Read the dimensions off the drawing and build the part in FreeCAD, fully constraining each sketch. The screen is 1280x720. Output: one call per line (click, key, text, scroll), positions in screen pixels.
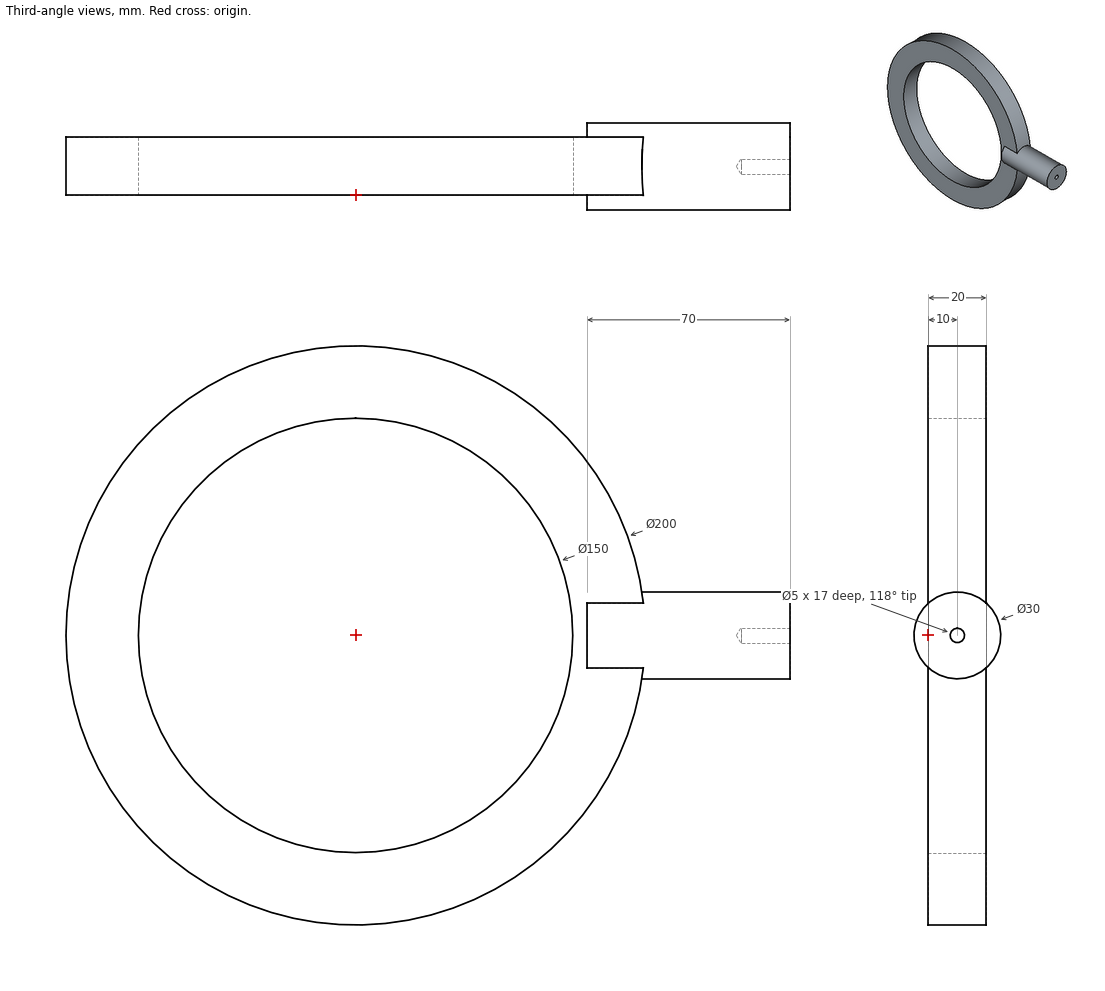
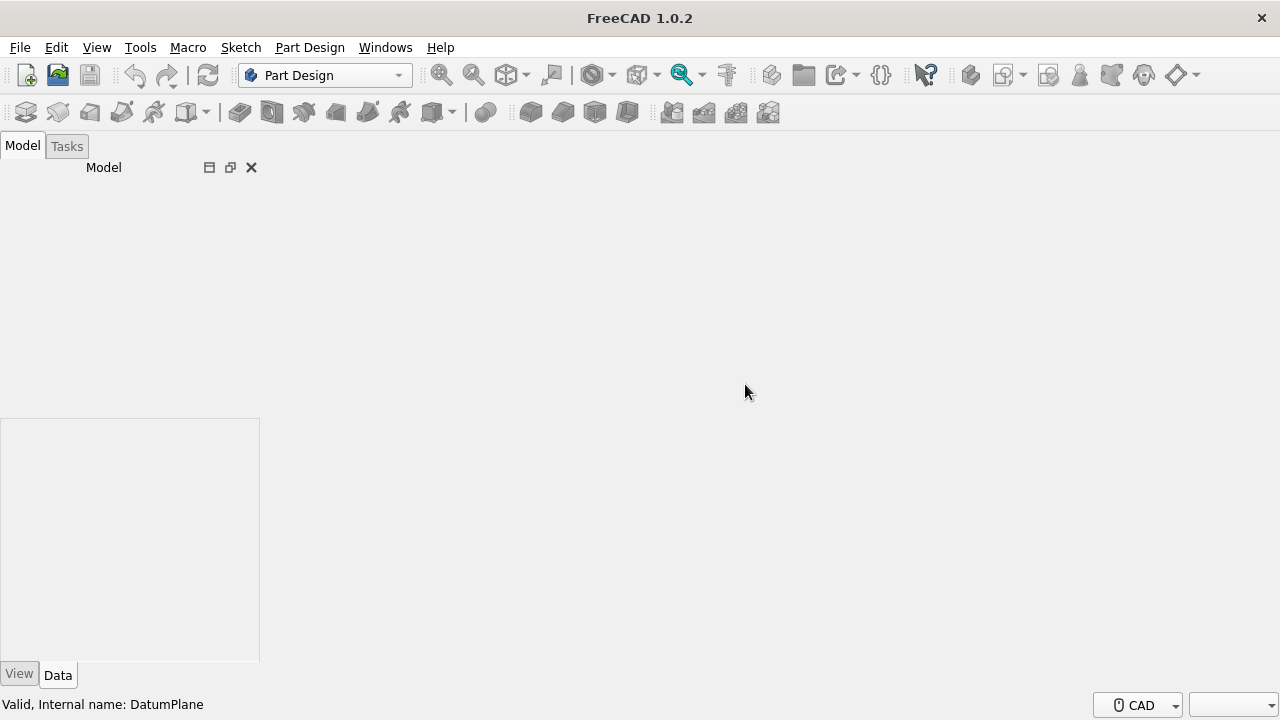
key(ctrl+n)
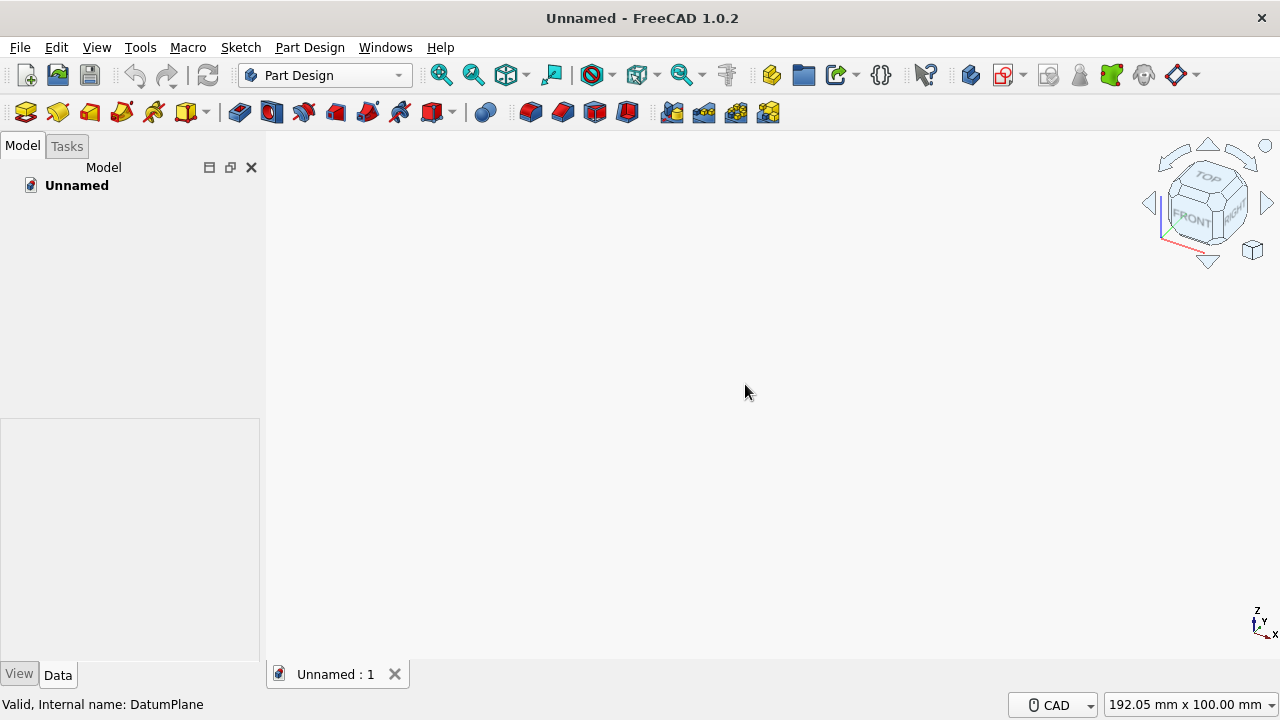
click(1004, 76)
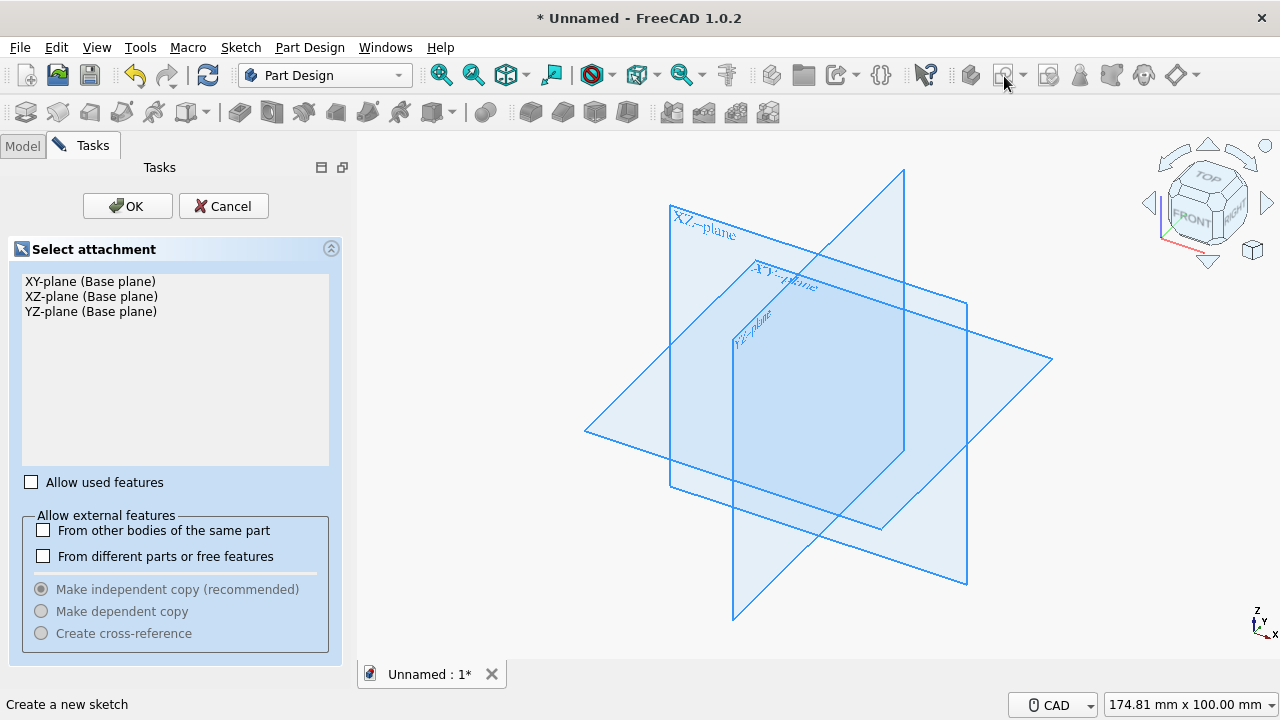
click(82, 296)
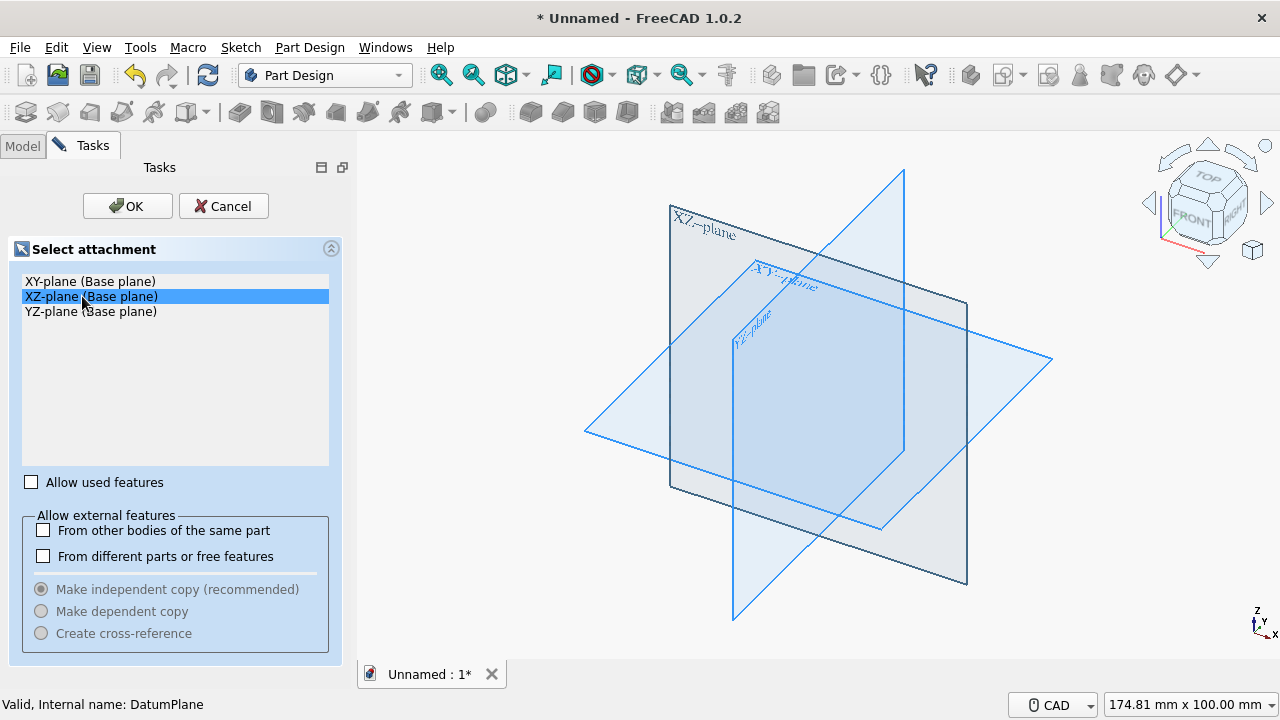
click(128, 206)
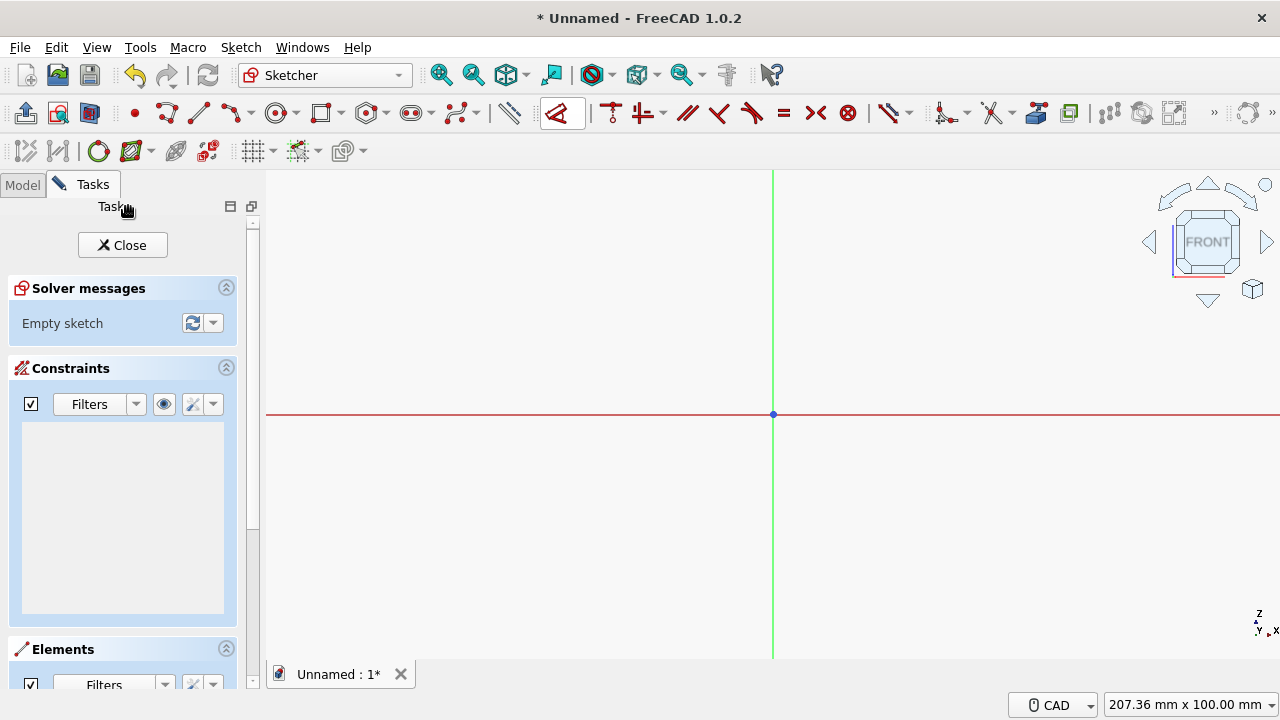
scroll(675, 414, down, 6)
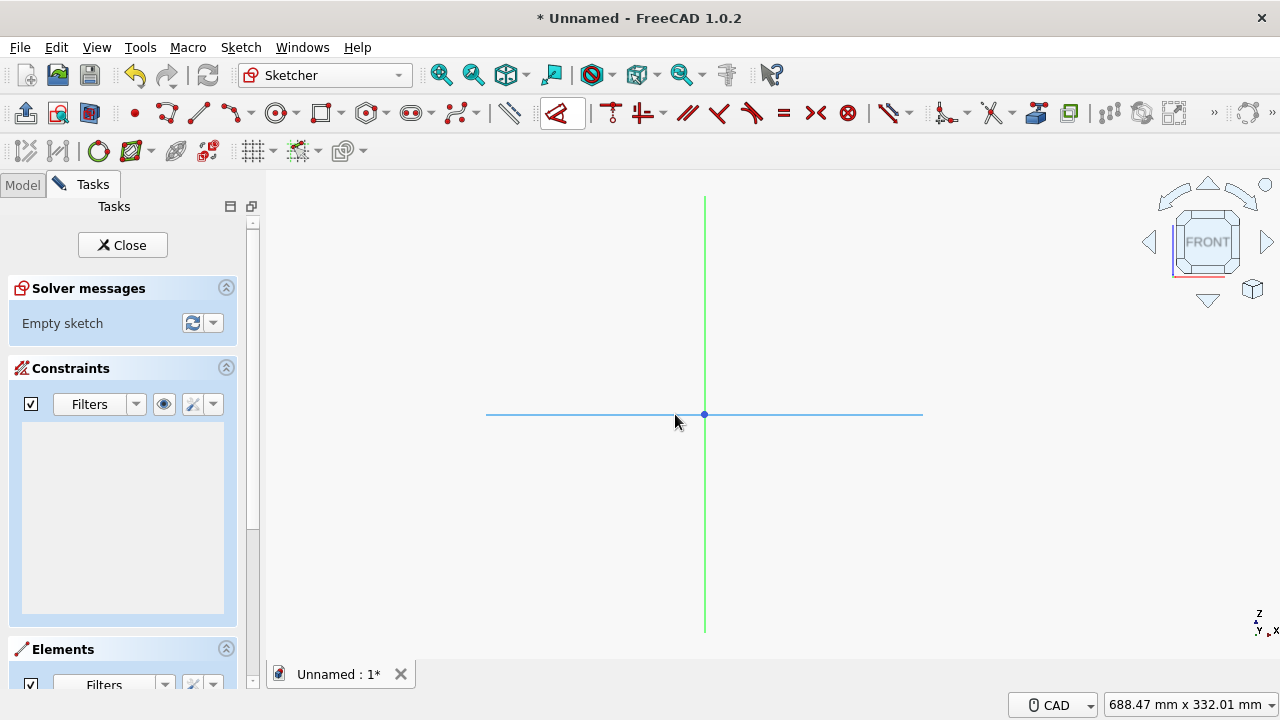
key(g)
key(c)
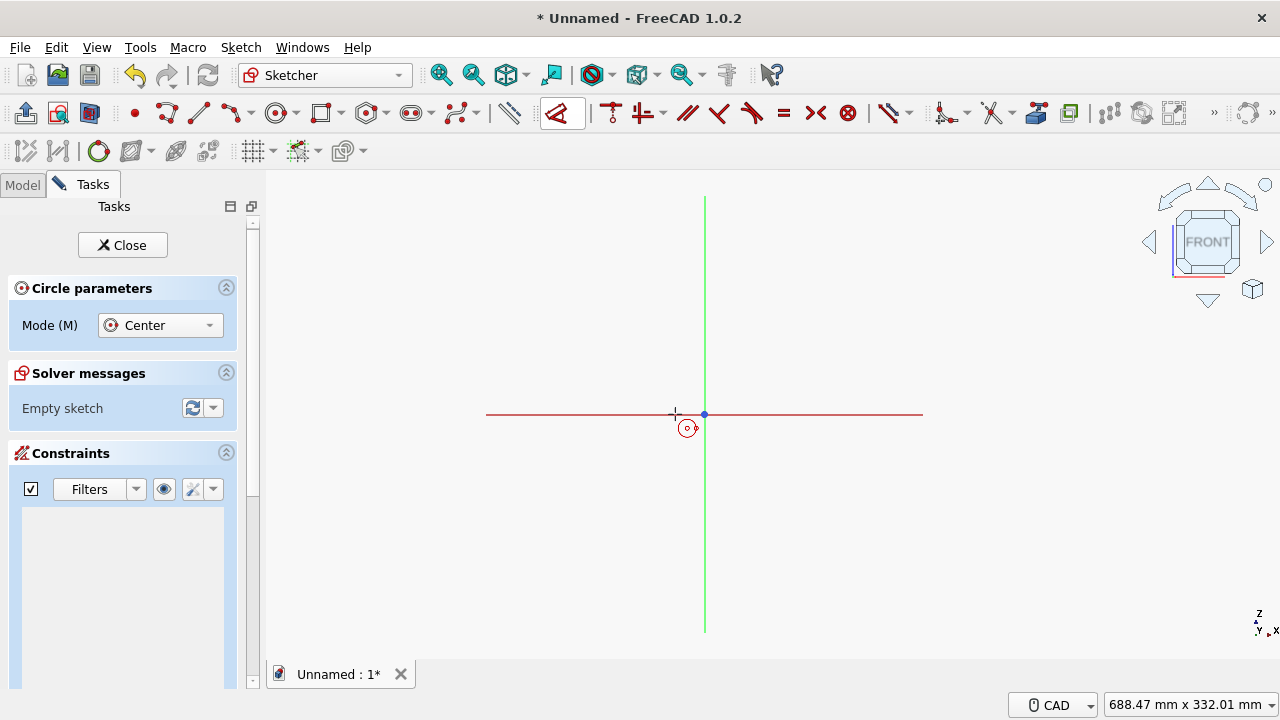
click(705, 414)
click(809, 310)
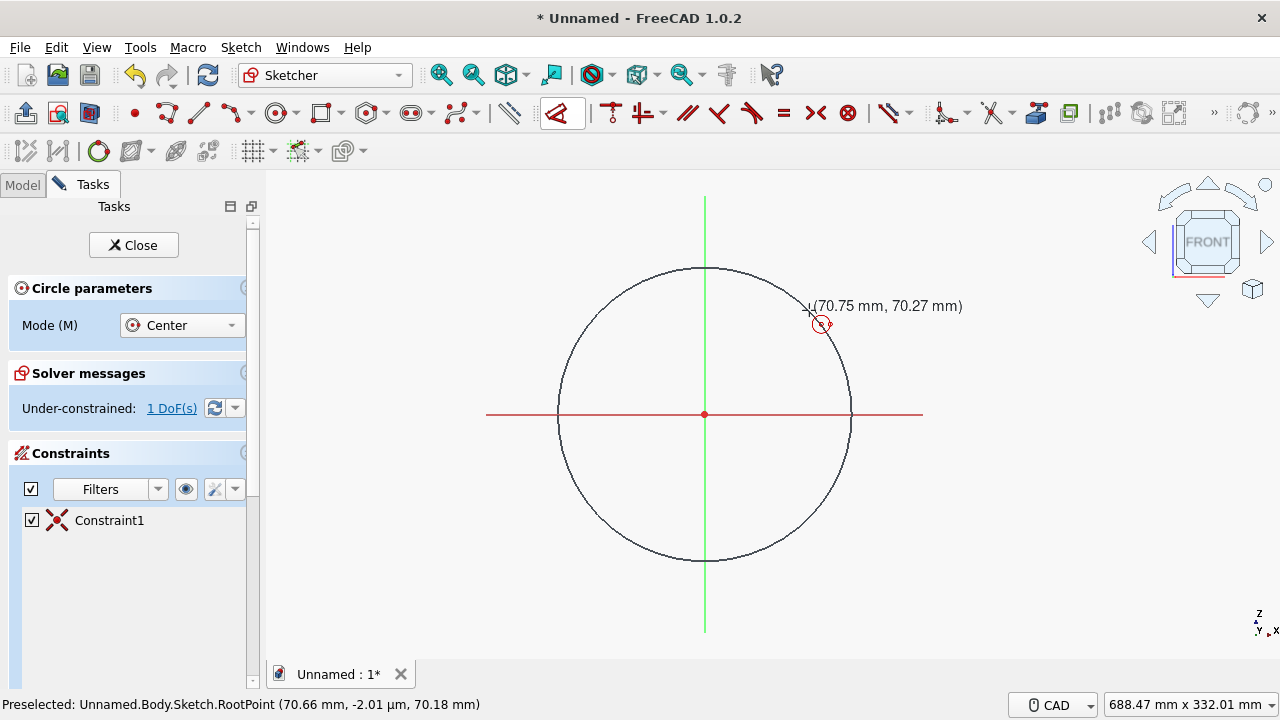
click(705, 414)
click(783, 336)
key(Escape)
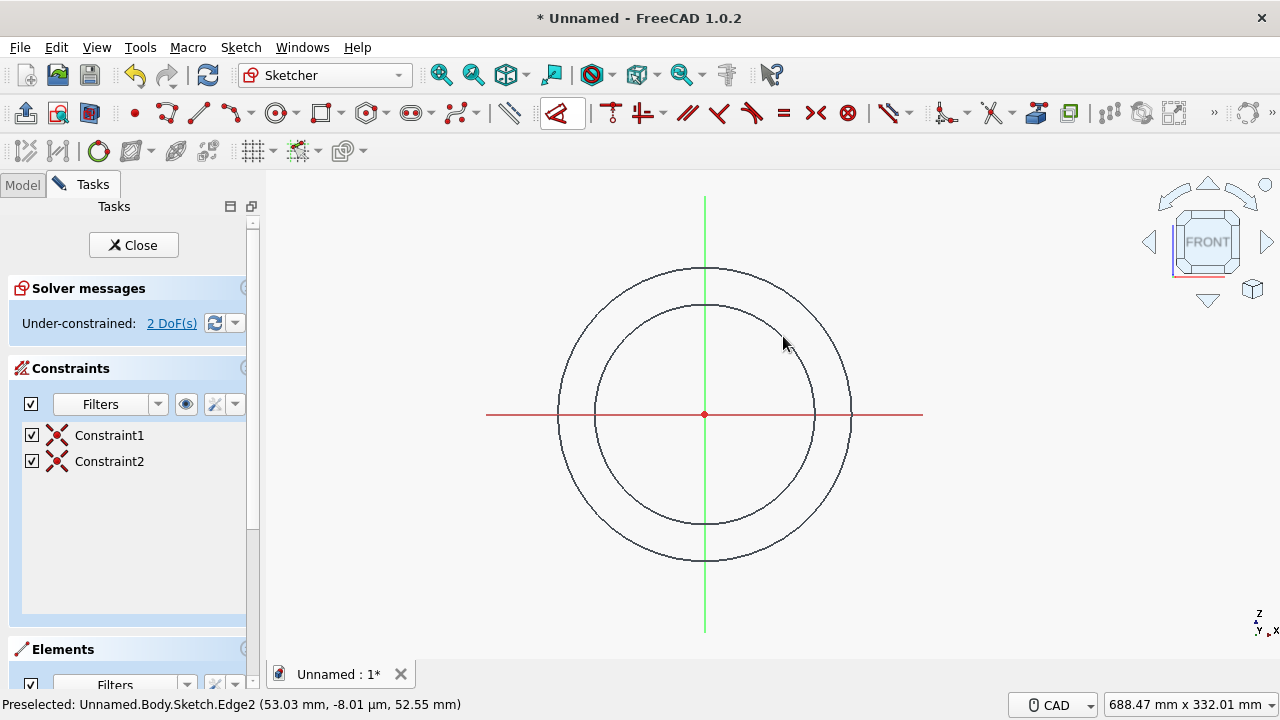
key(d)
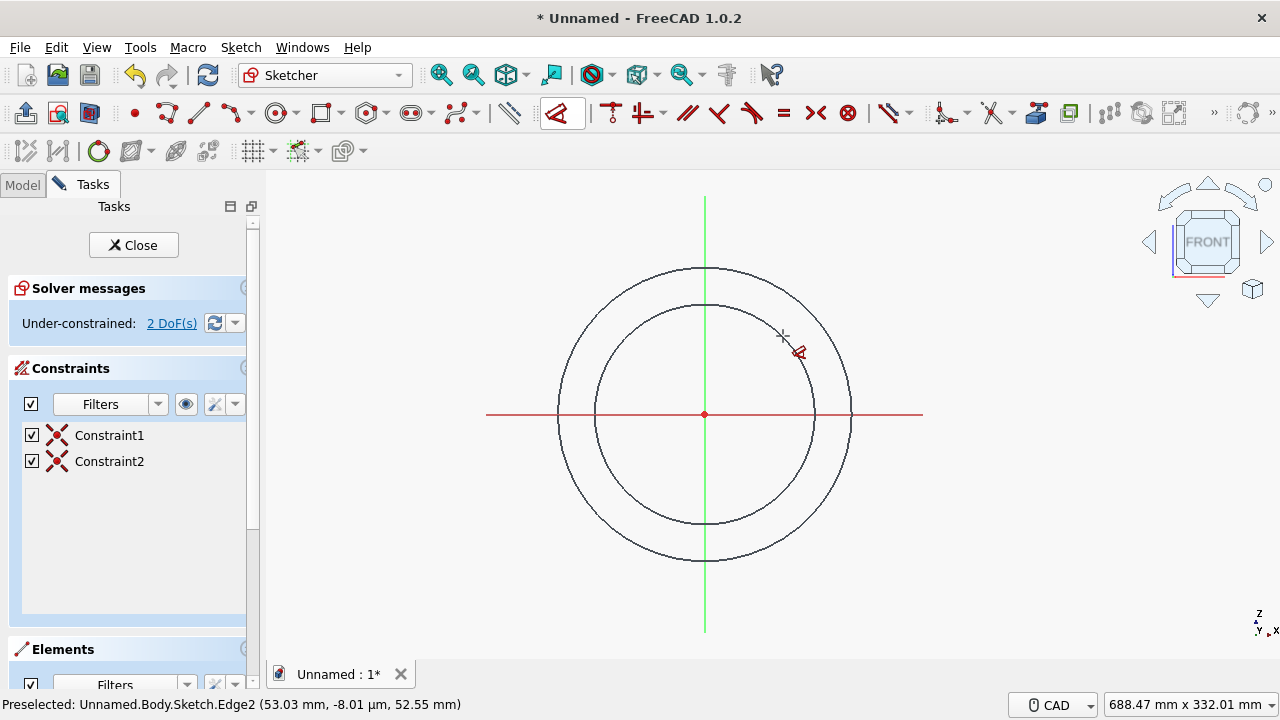
click(808, 310)
click(830, 287)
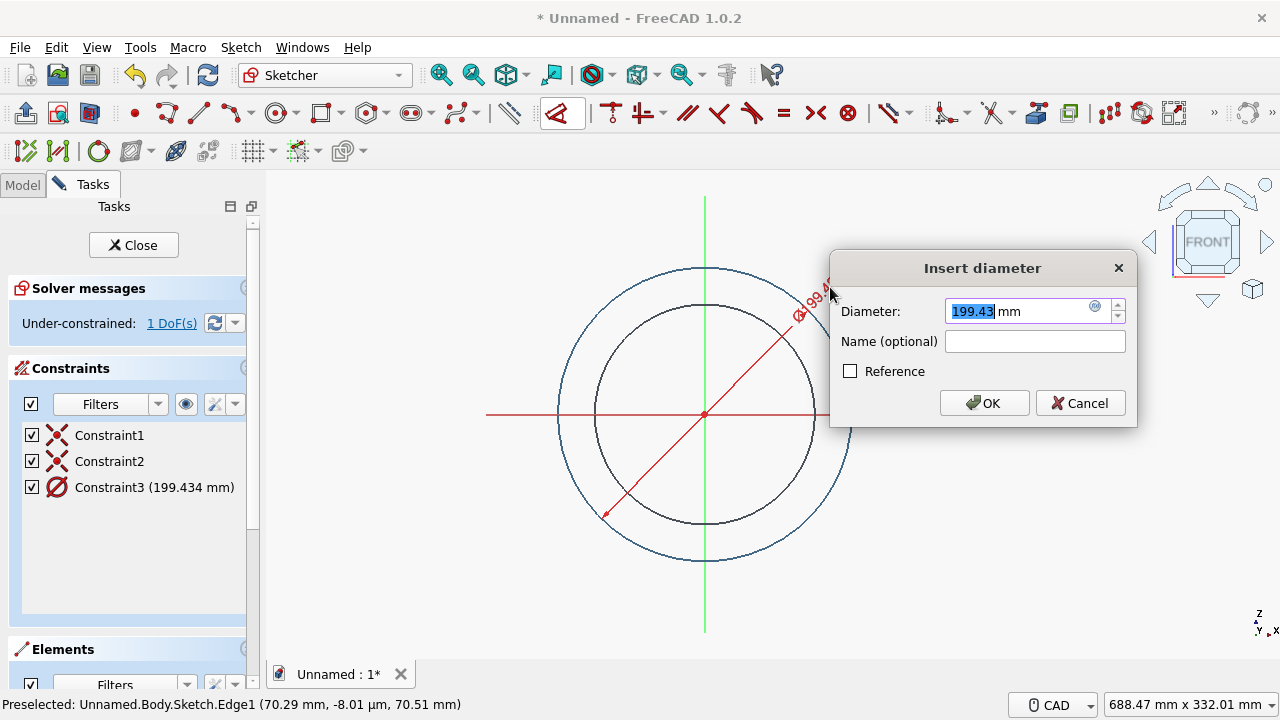
text(200)
key(Return)